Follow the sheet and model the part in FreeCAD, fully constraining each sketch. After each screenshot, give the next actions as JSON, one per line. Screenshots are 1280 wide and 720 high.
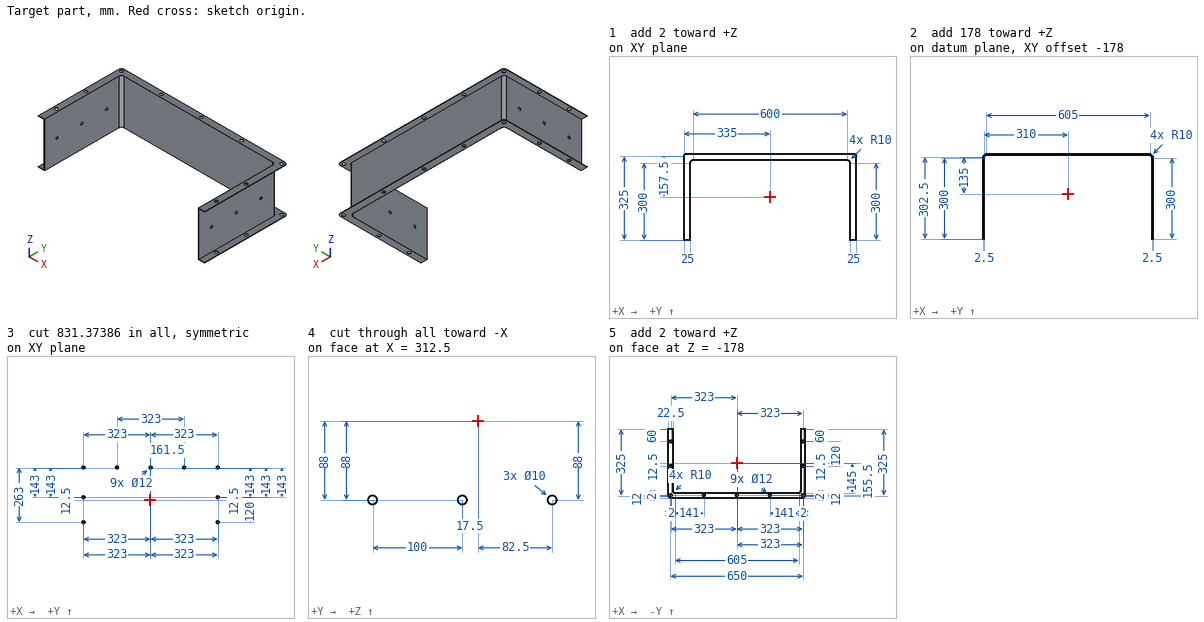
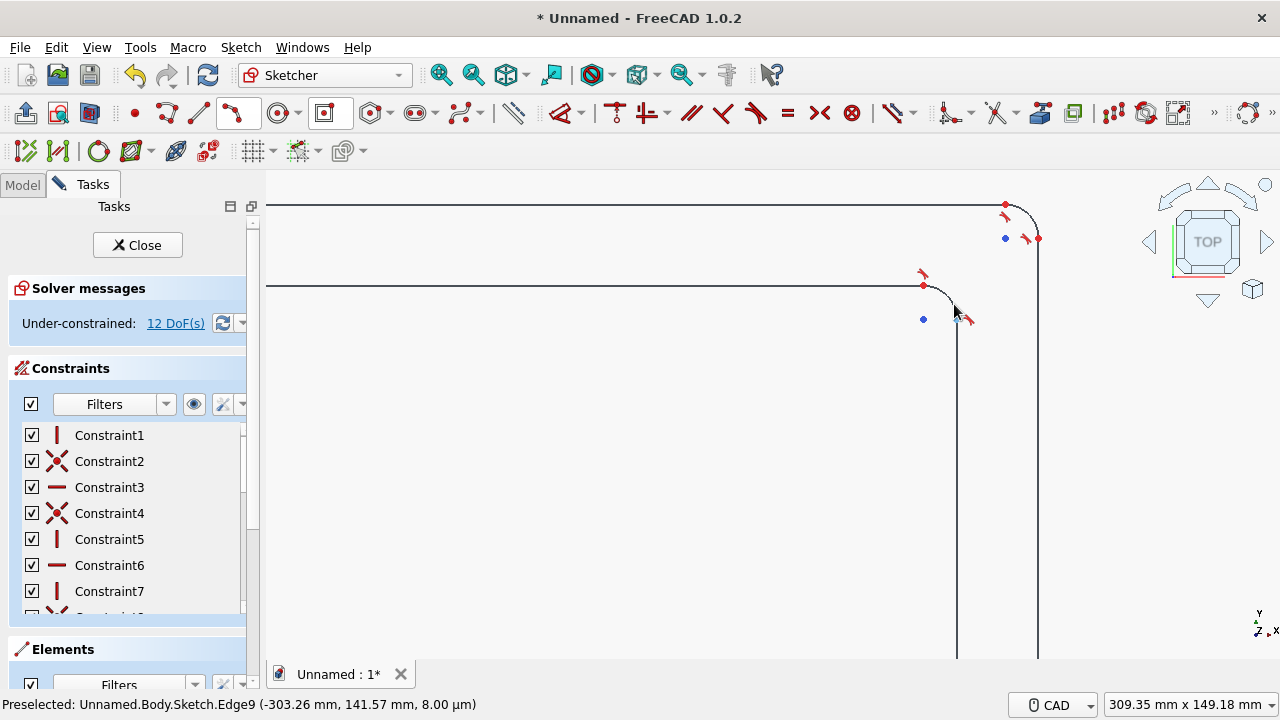
{"action": "left_click", "coordinate": [953, 304]}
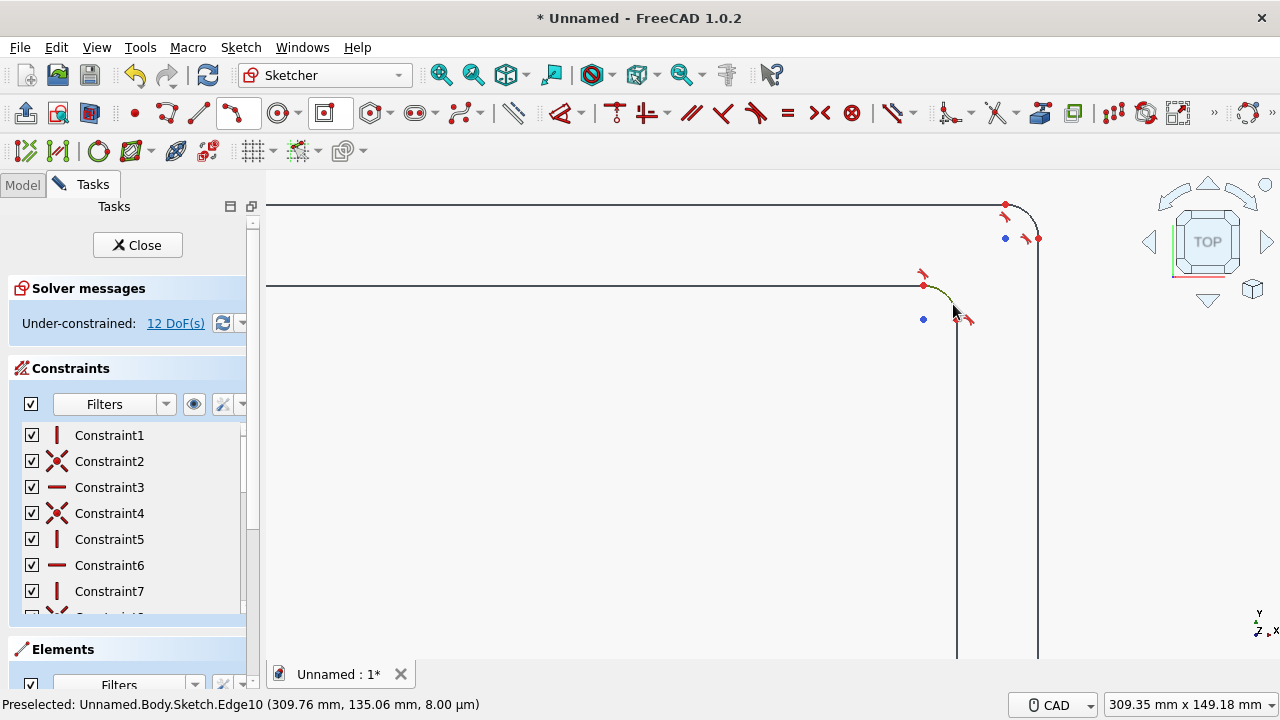
{"action": "left_click", "coordinate": [1035, 223]}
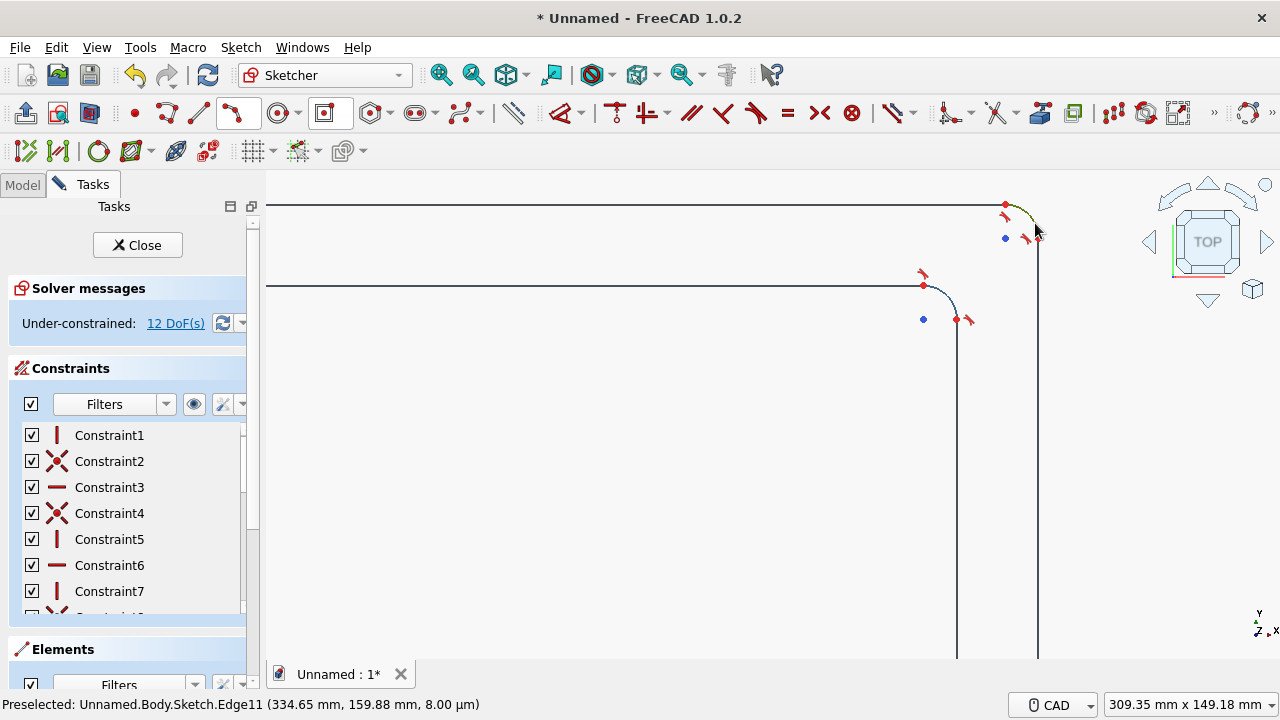
{"action": "scroll", "coordinate": [955, 304], "scroll_direction": "down", "scroll_amount": 7}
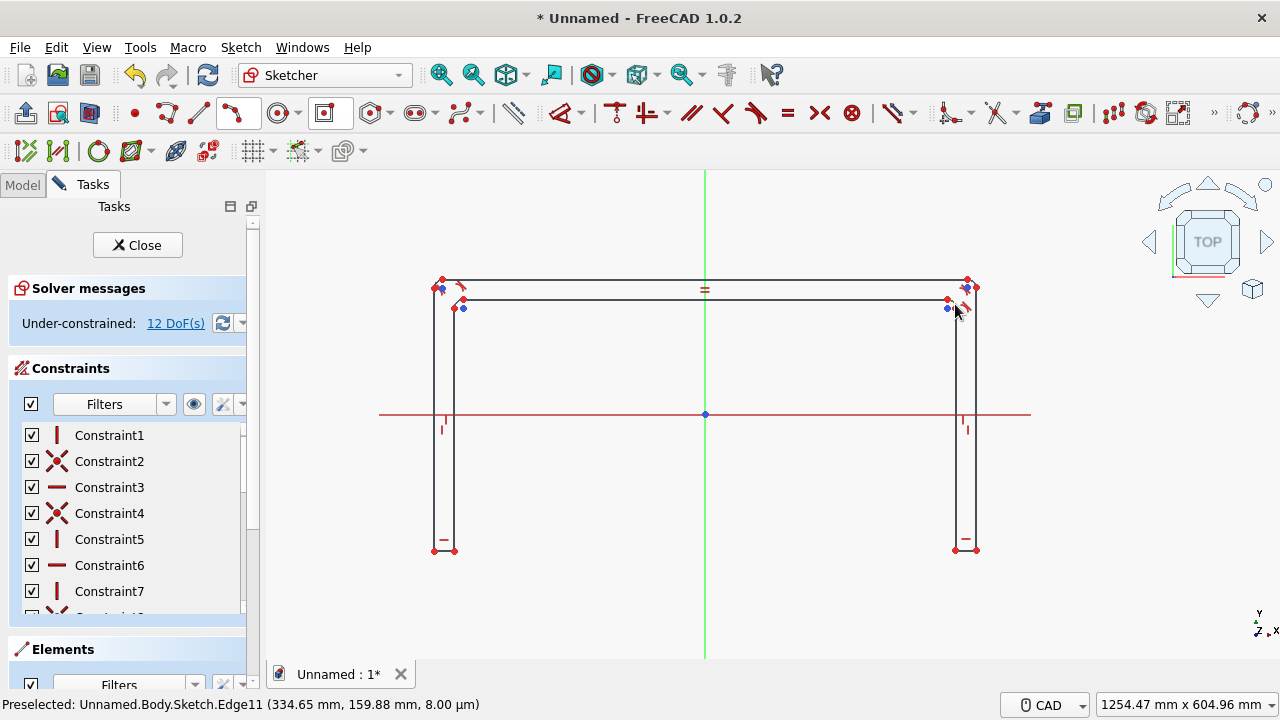
{"action": "scroll", "coordinate": [439, 281], "scroll_direction": "up", "scroll_amount": 7}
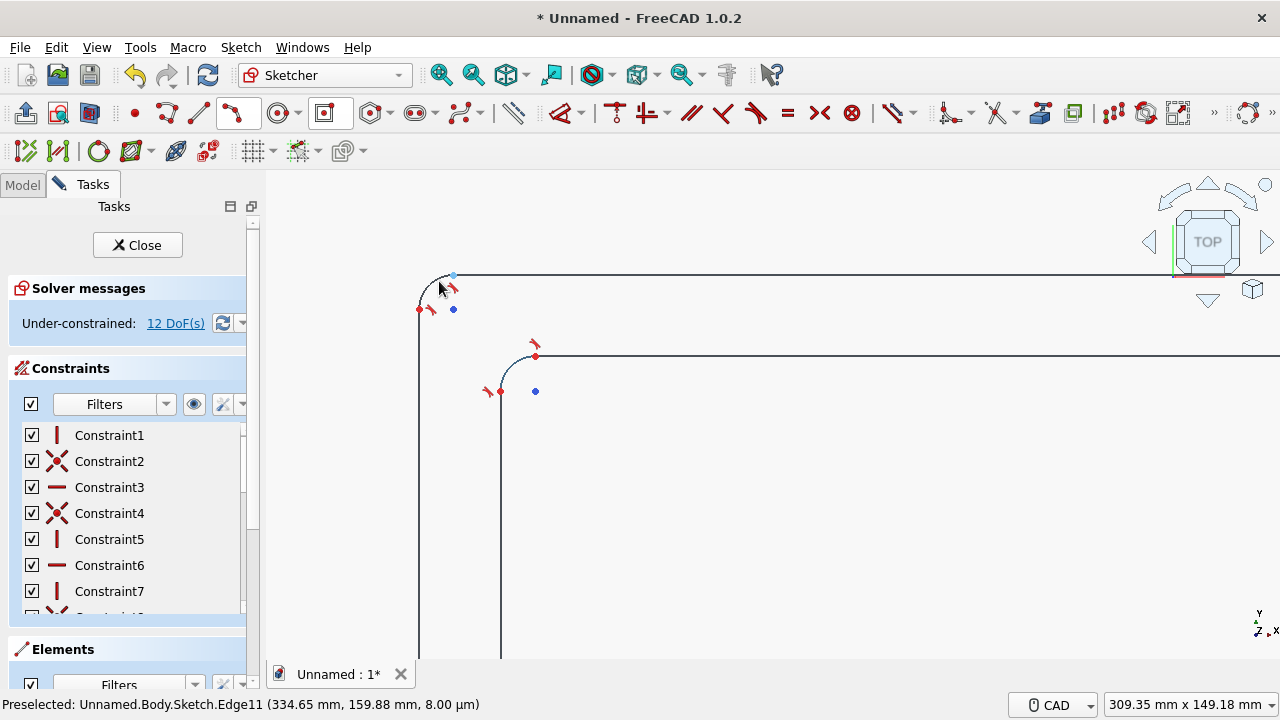
{"action": "left_click", "coordinate": [438, 279]}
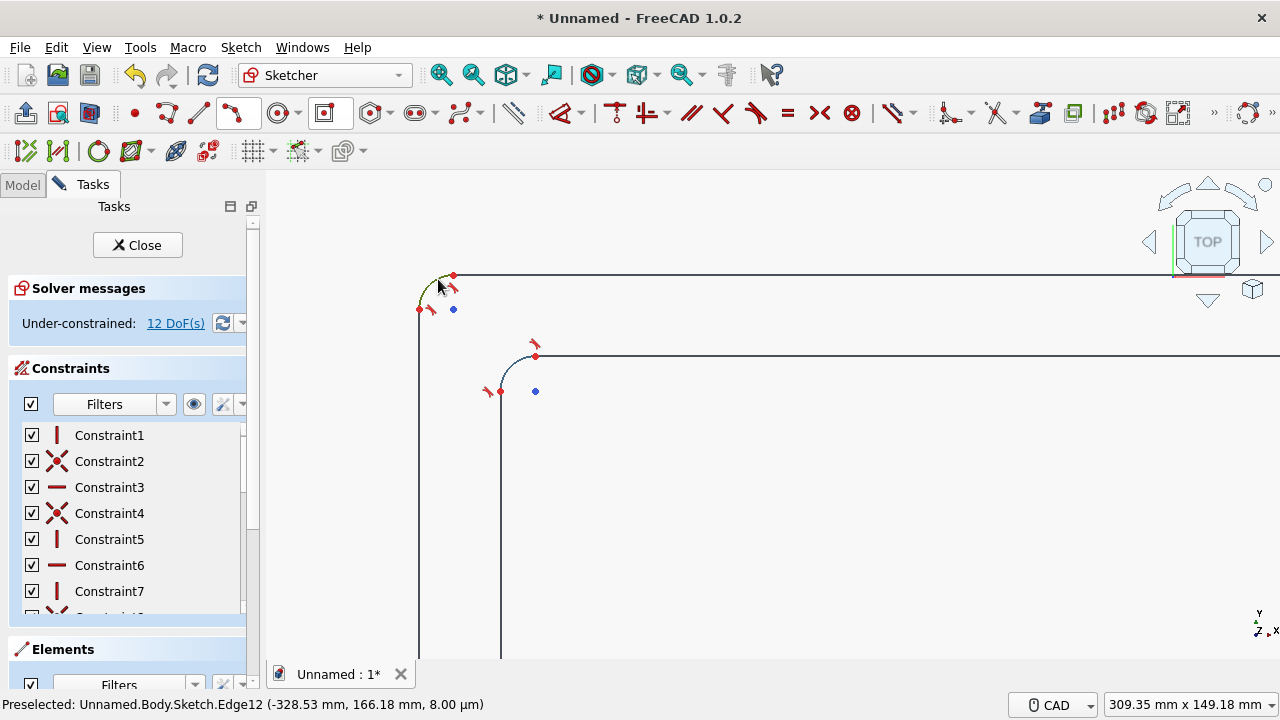
{"action": "left_click", "coordinate": [788, 114]}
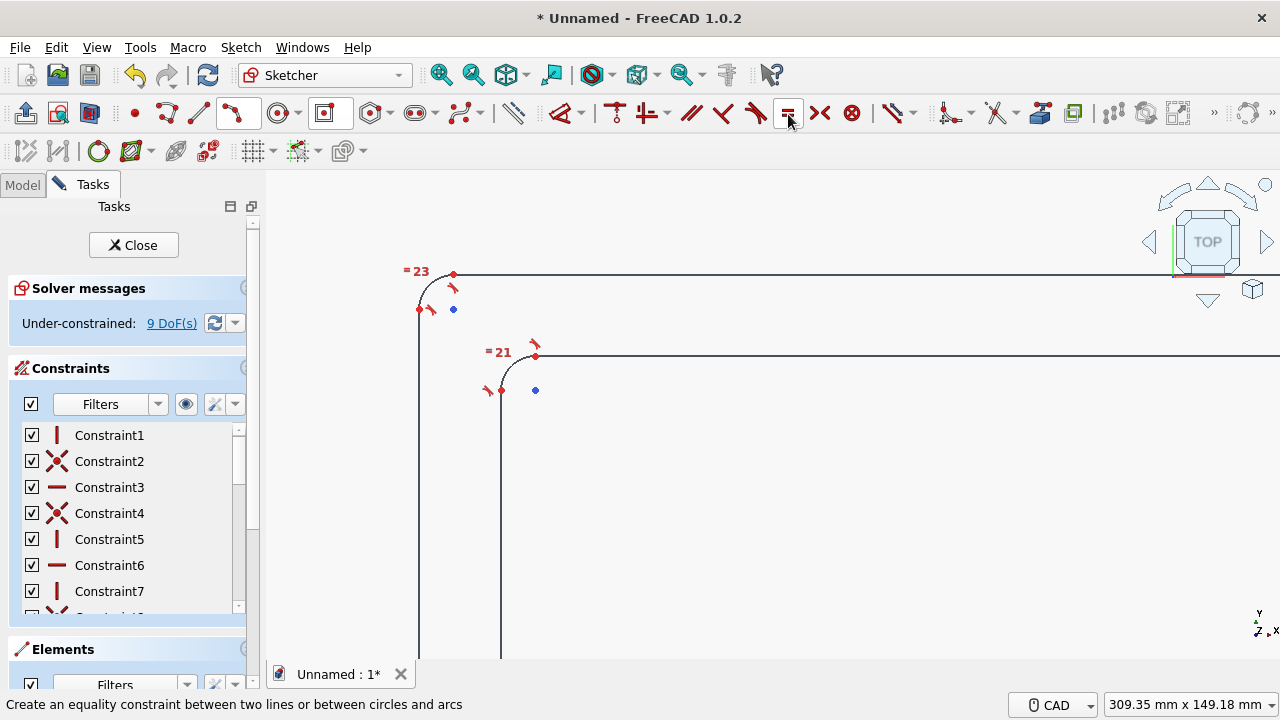
{"action": "left_click", "coordinate": [560, 114]}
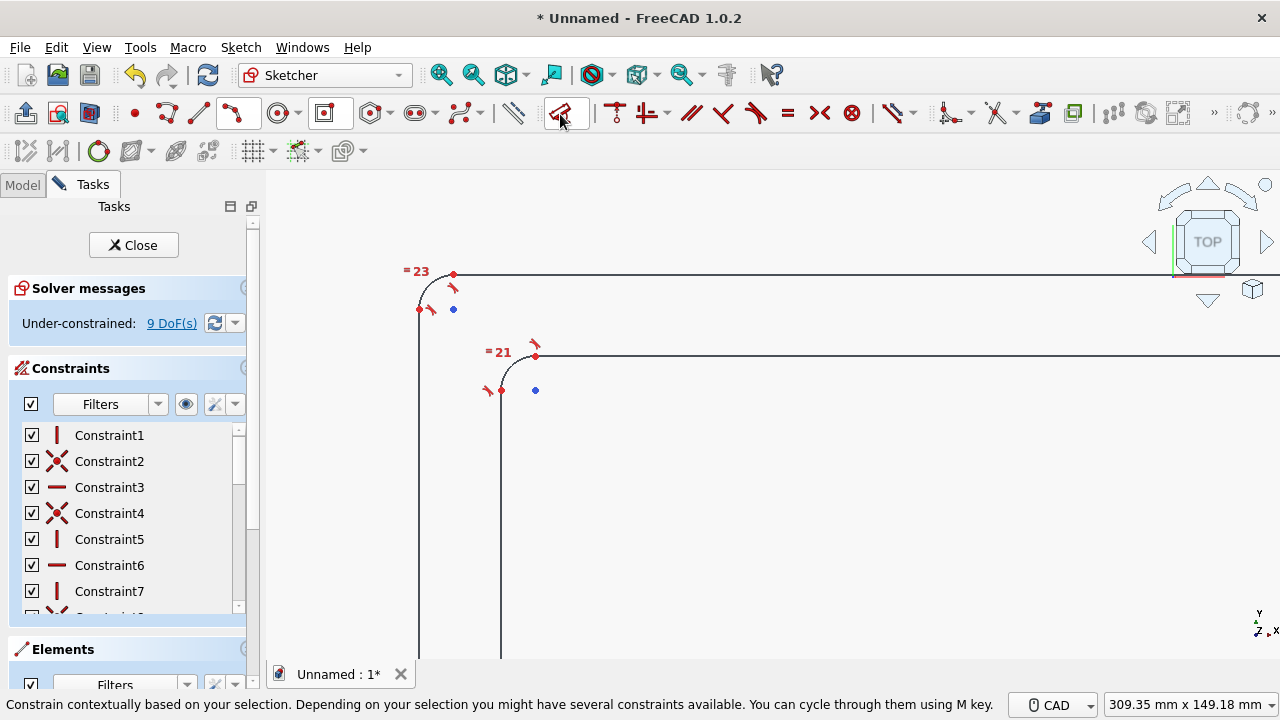
{"action": "left_click", "coordinate": [520, 360]}
{"action": "left_click", "coordinate": [505, 332]}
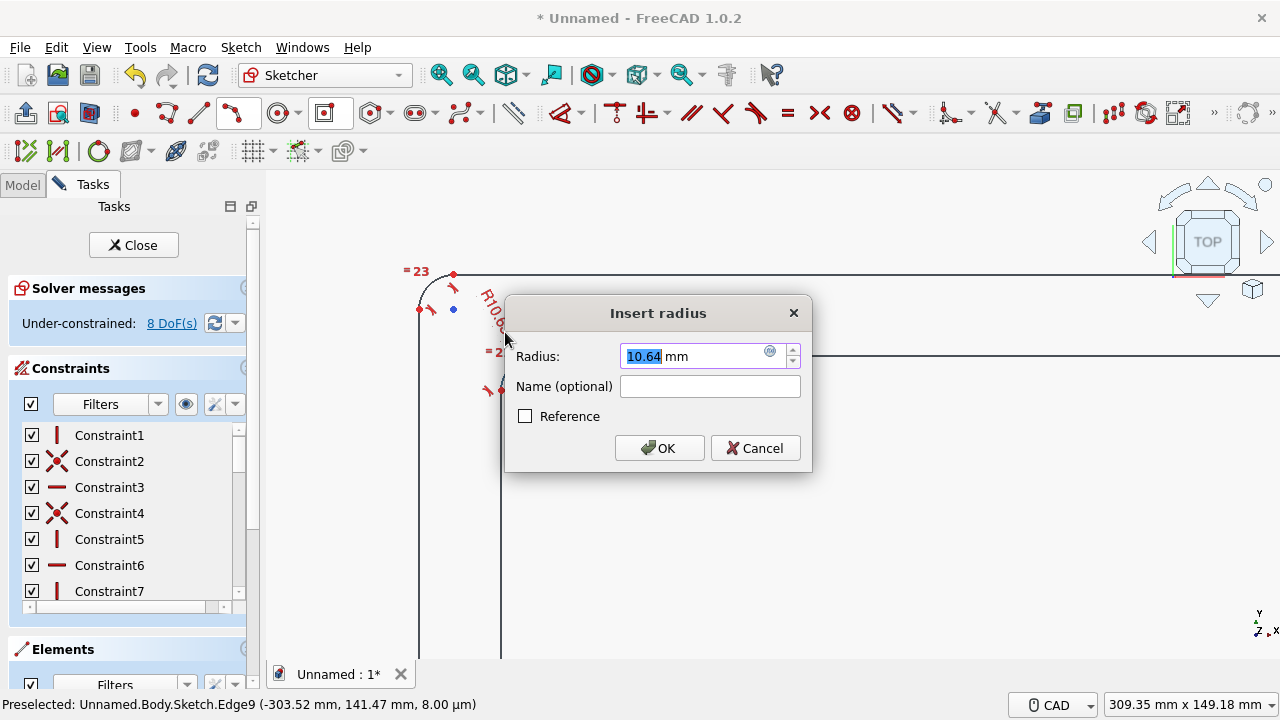
{"action": "type", "text": "10"}
{"action": "key", "text": "Return"}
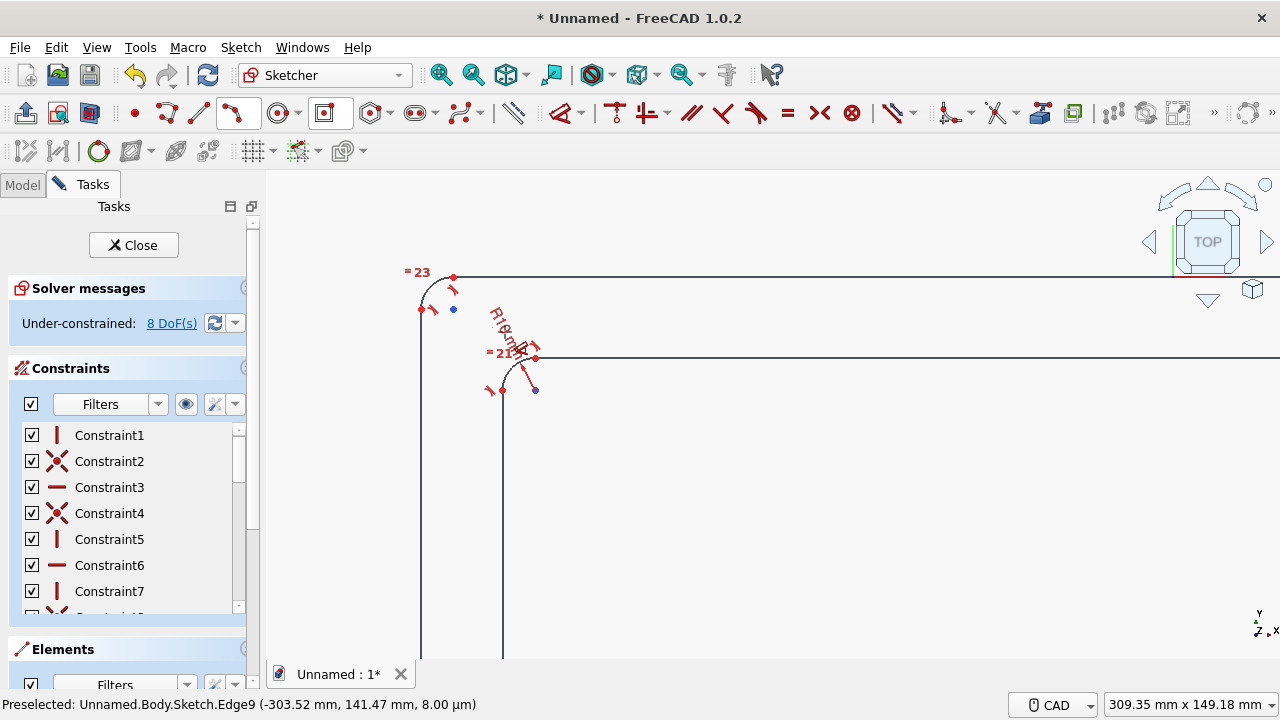
{"action": "scroll", "coordinate": [438, 281], "scroll_direction": "down", "scroll_amount": 7}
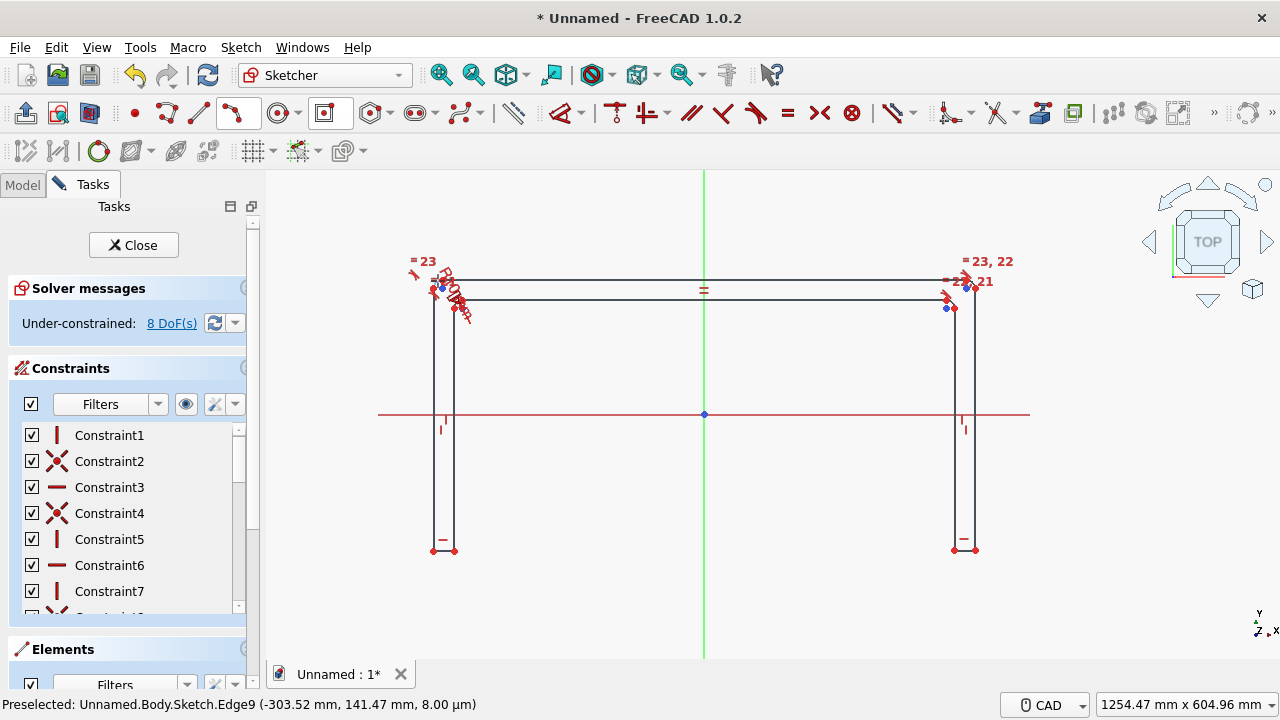
{"action": "scroll", "coordinate": [440, 551], "scroll_direction": "up", "scroll_amount": 5}